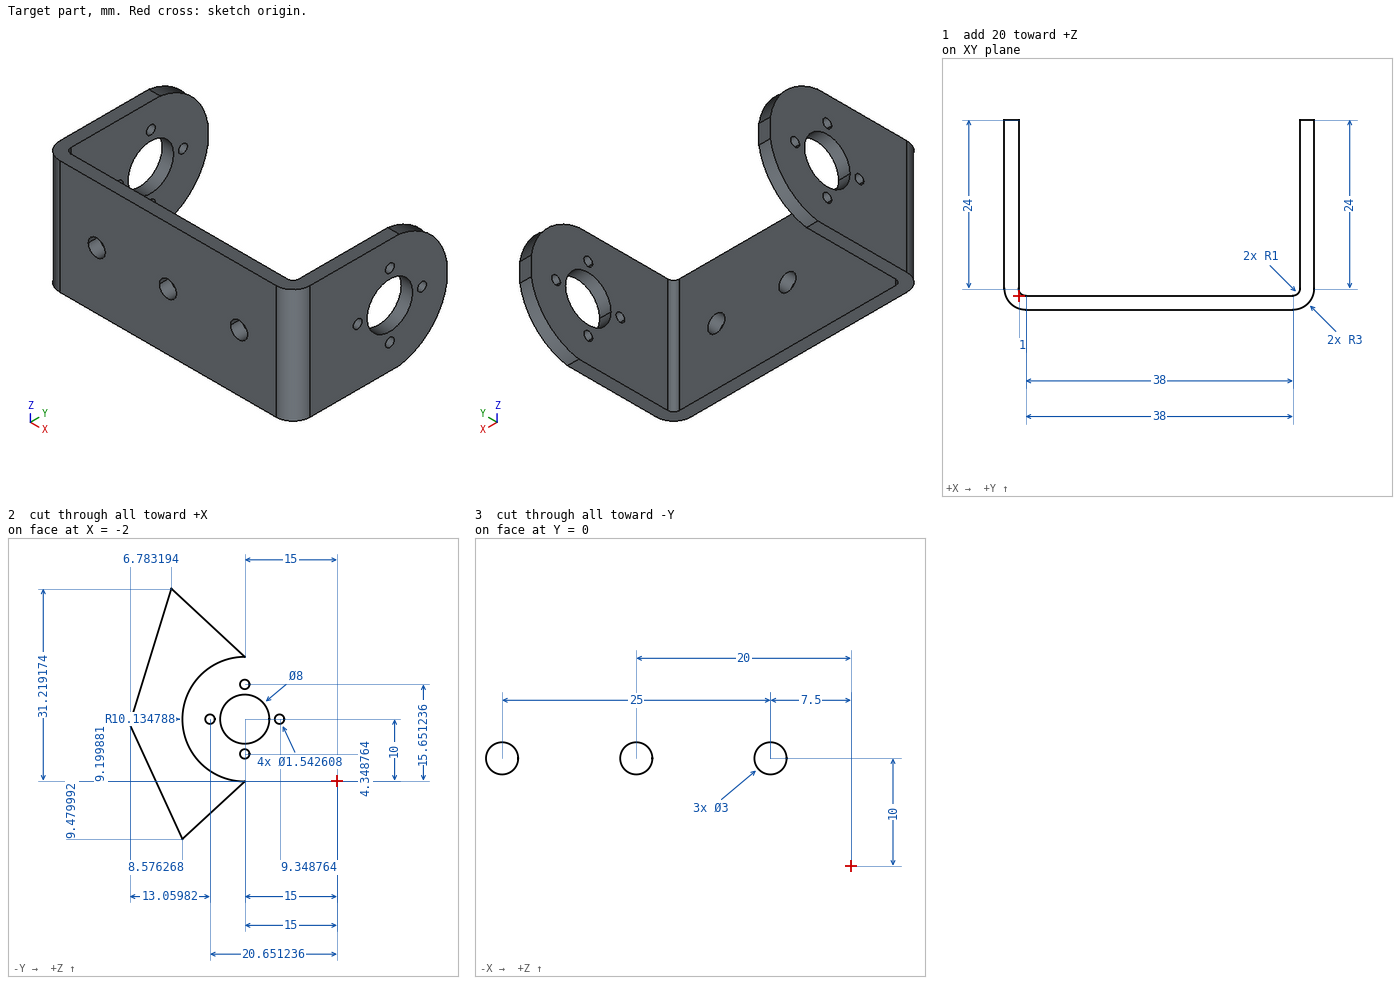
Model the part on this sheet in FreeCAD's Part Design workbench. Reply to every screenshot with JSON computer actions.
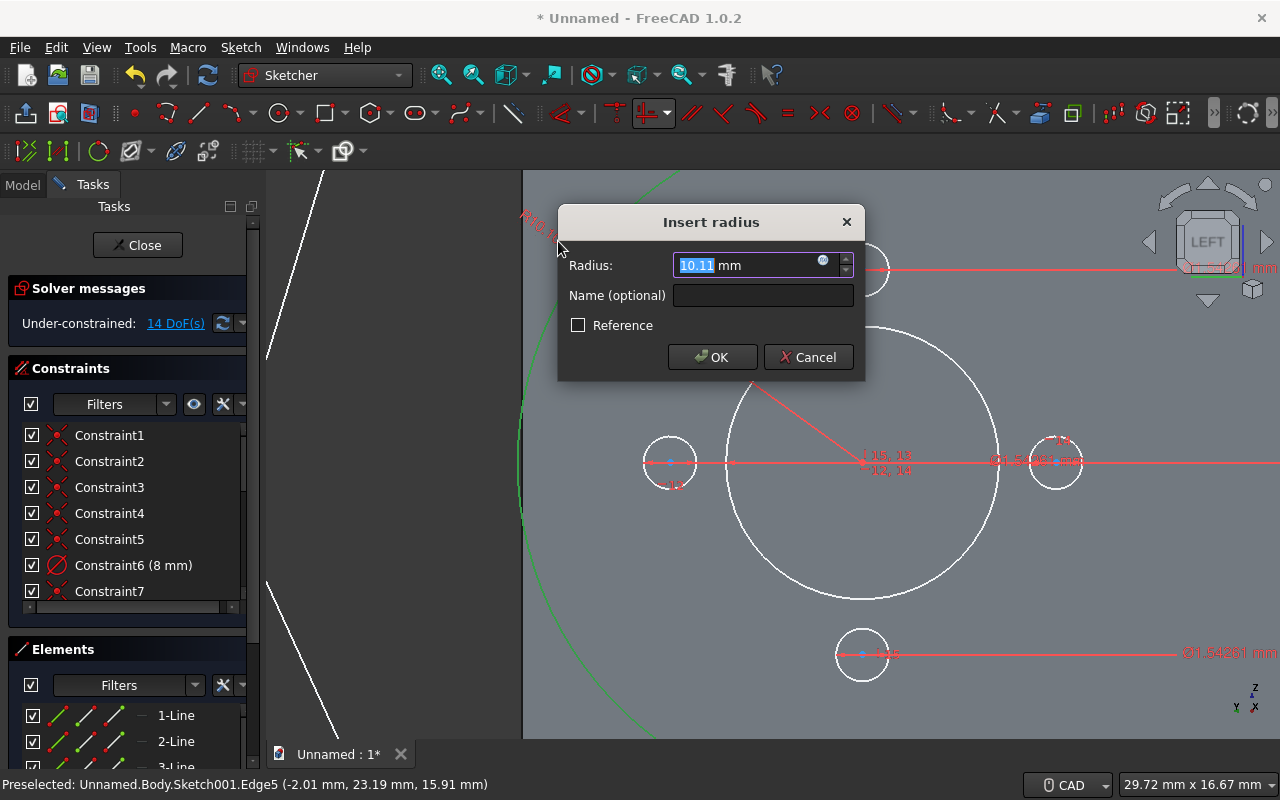
{"action": "type", "text": "10.134788"}
{"action": "key", "text": "Return"}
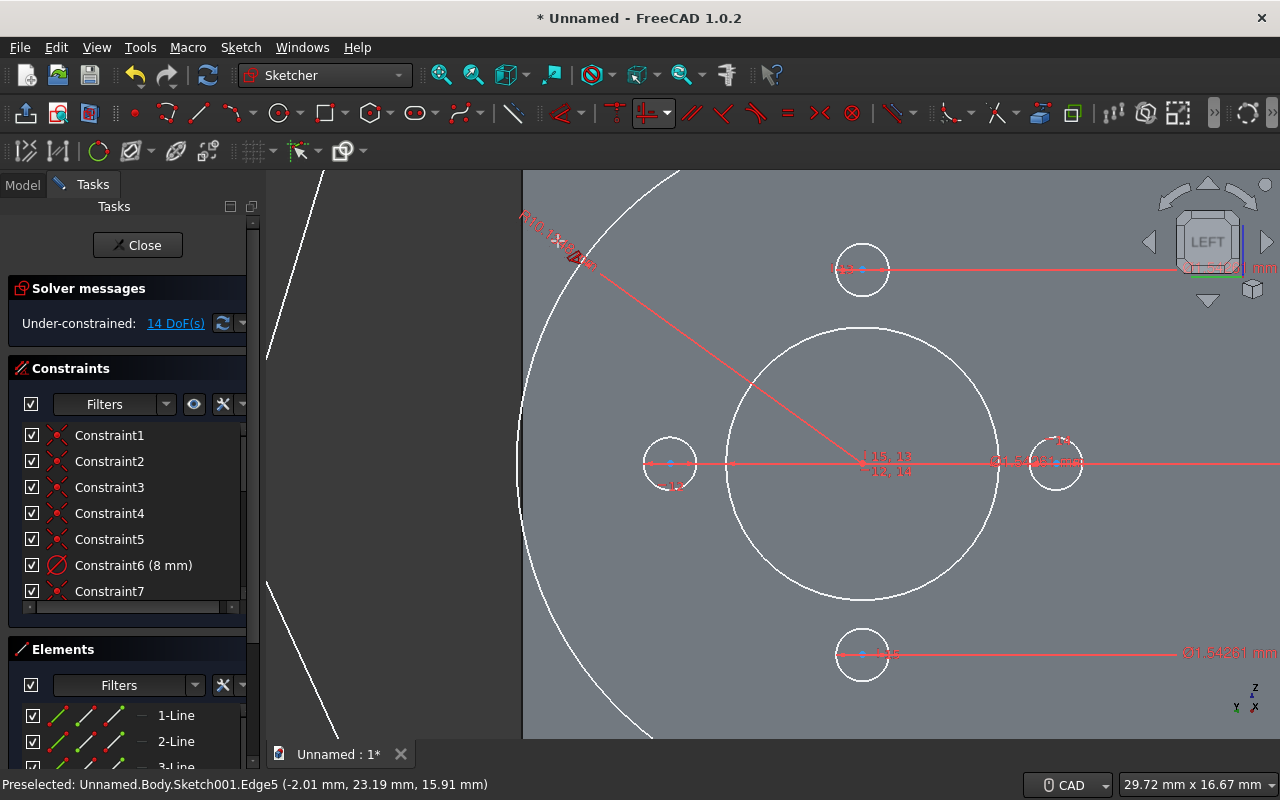
{"action": "left_click", "coordinate": [863, 464]}
{"action": "left_click", "coordinate": [931, 430]}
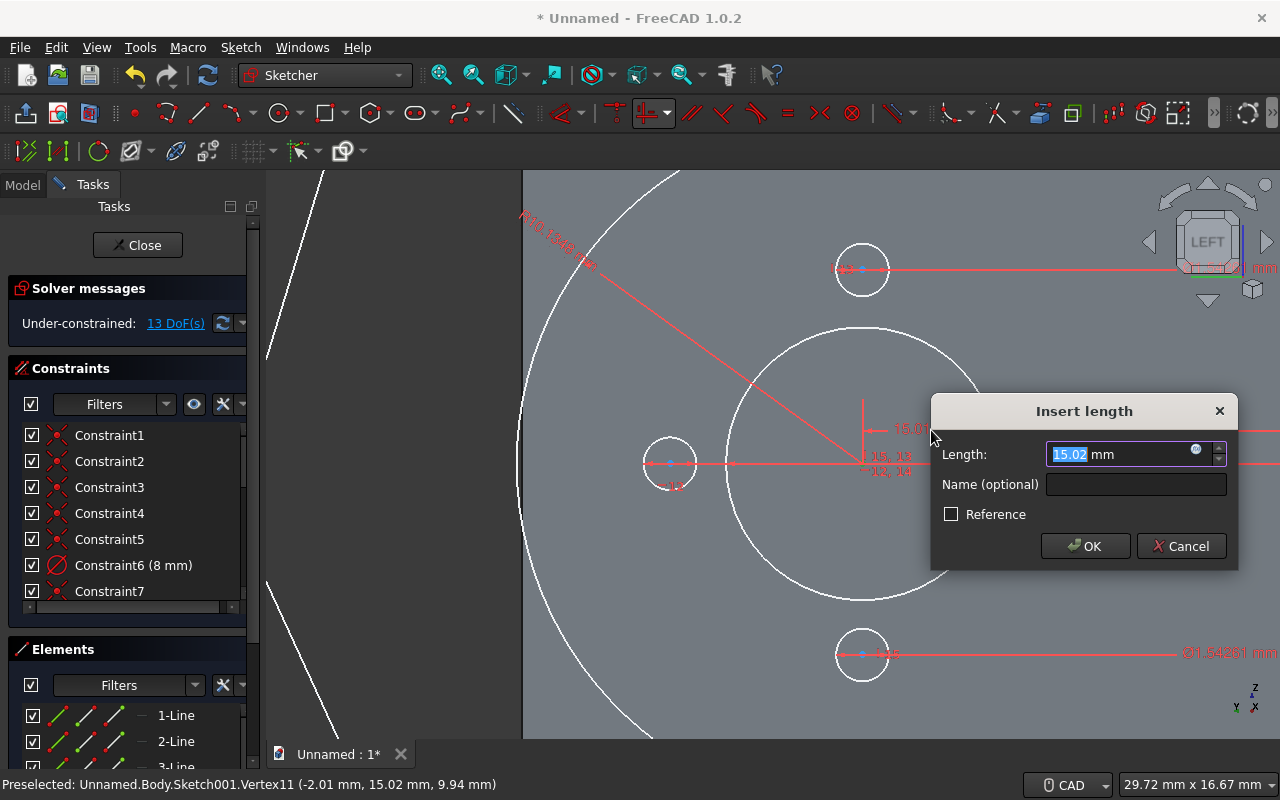
{"action": "type", "text": "15"}
{"action": "key", "text": "Return"}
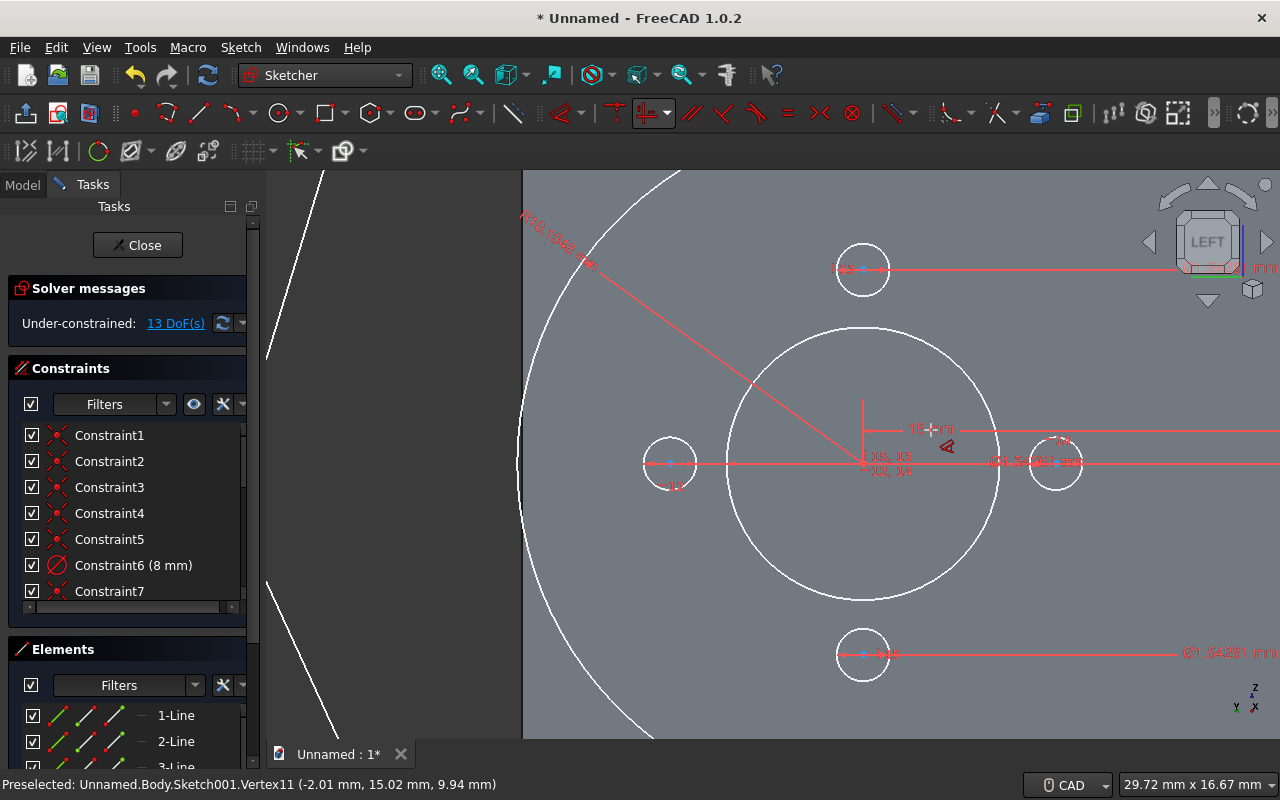
{"action": "left_click", "coordinate": [863, 464]}
{"action": "left_click", "coordinate": [829, 531]}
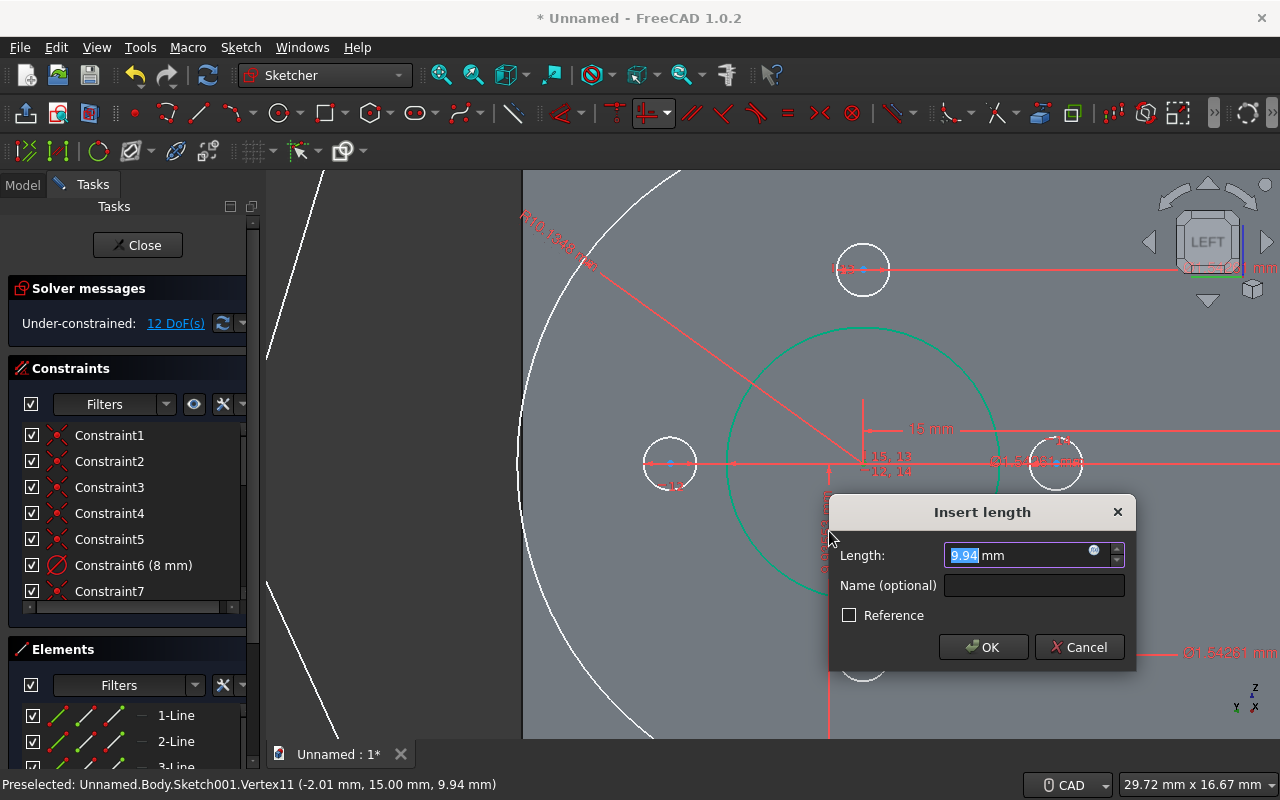
{"action": "type", "text": "10"}
{"action": "key", "text": "Return"}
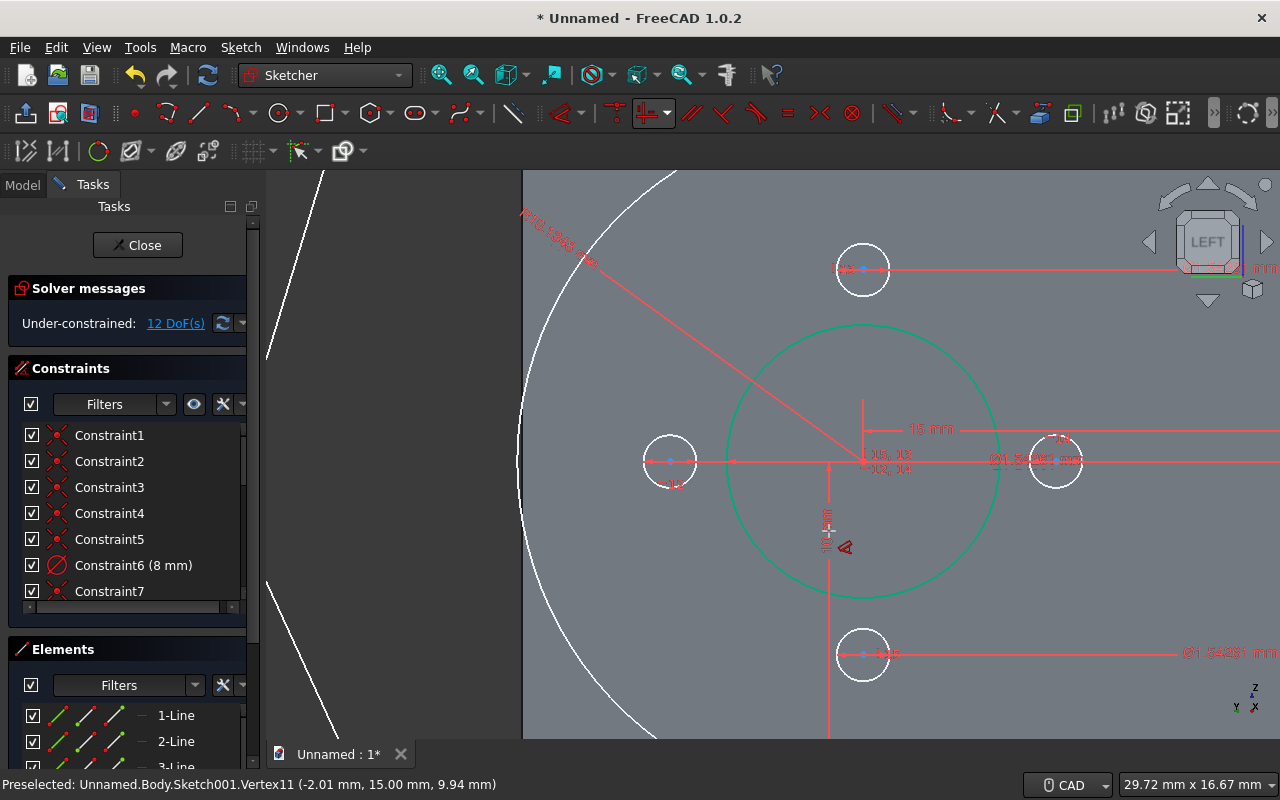
{"action": "scroll", "coordinate": [673, 462], "scroll_direction": "down", "scroll_amount": 7}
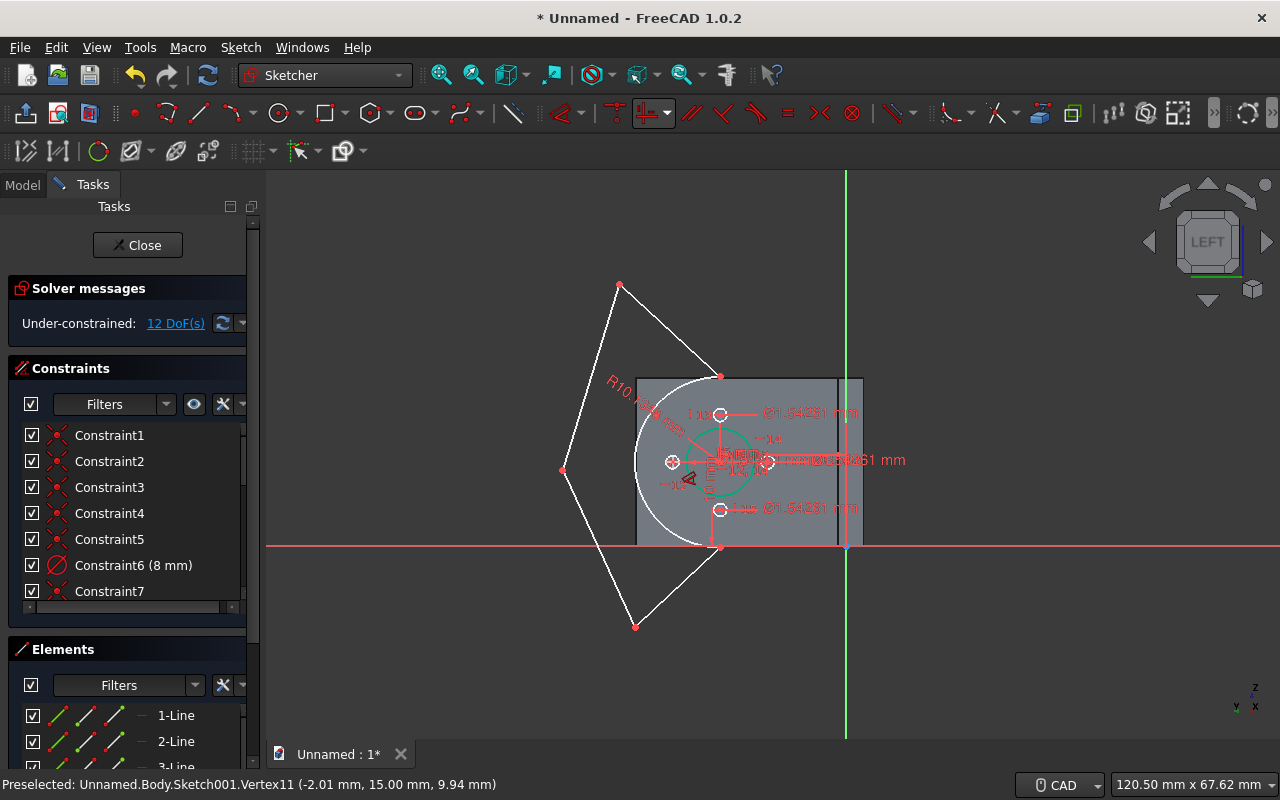
{"action": "left_click", "coordinate": [720, 377]}
{"action": "left_click", "coordinate": [783, 580]}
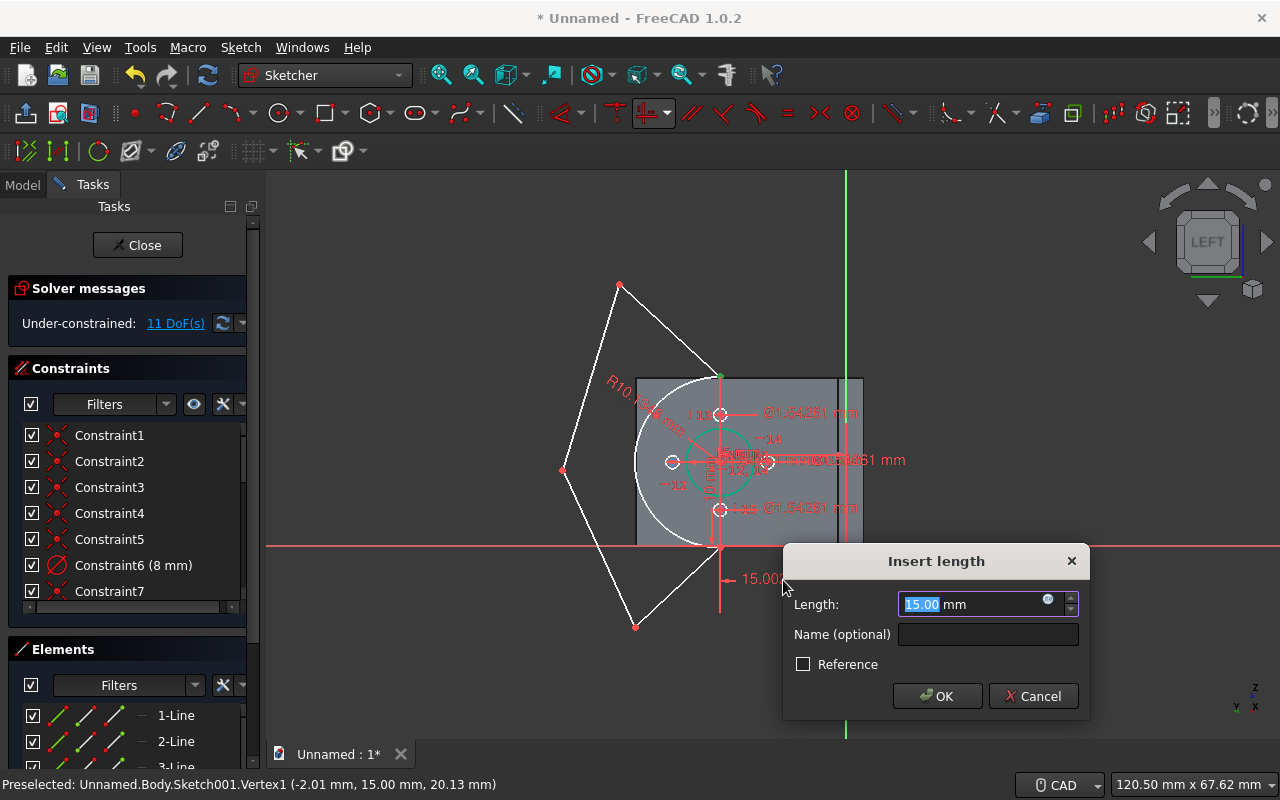
{"action": "type", "text": "15"}
{"action": "key", "text": "Return"}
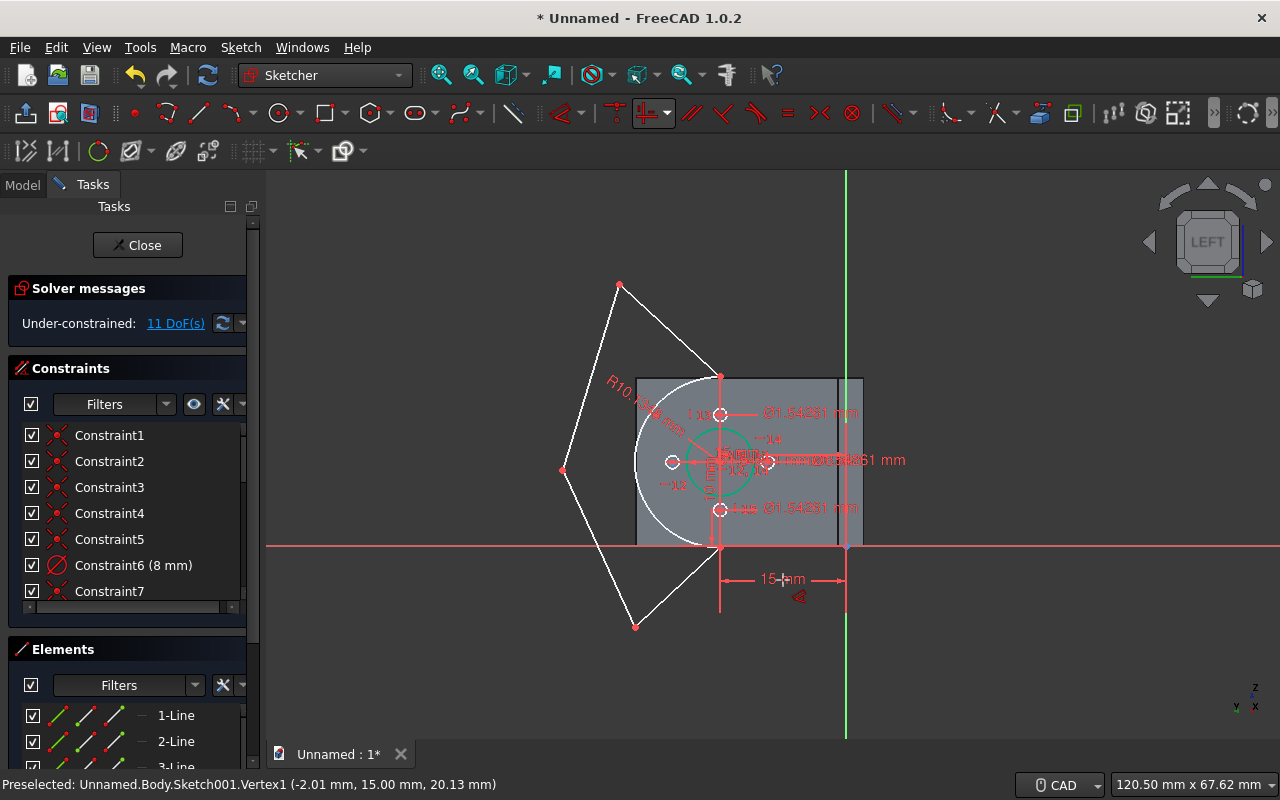
{"action": "left_click", "coordinate": [720, 548]}
{"action": "left_click", "coordinate": [783, 512]}